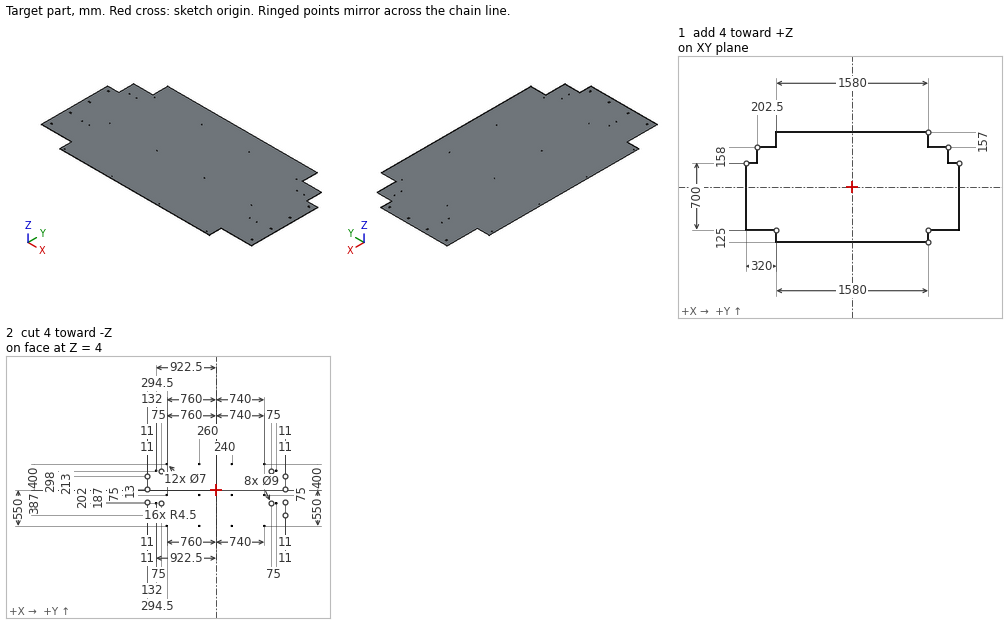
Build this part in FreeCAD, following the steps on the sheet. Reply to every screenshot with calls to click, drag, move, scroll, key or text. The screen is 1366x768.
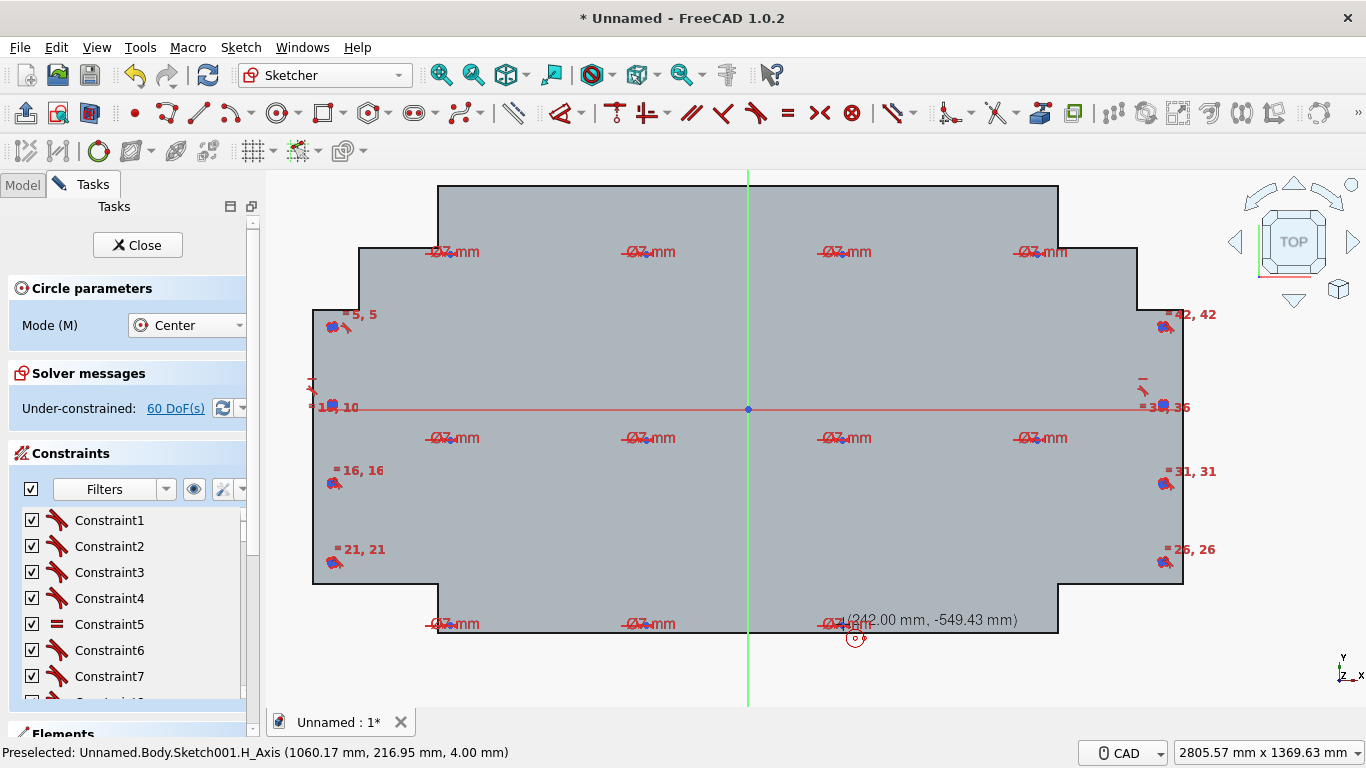
scroll(1038, 625, up, 15)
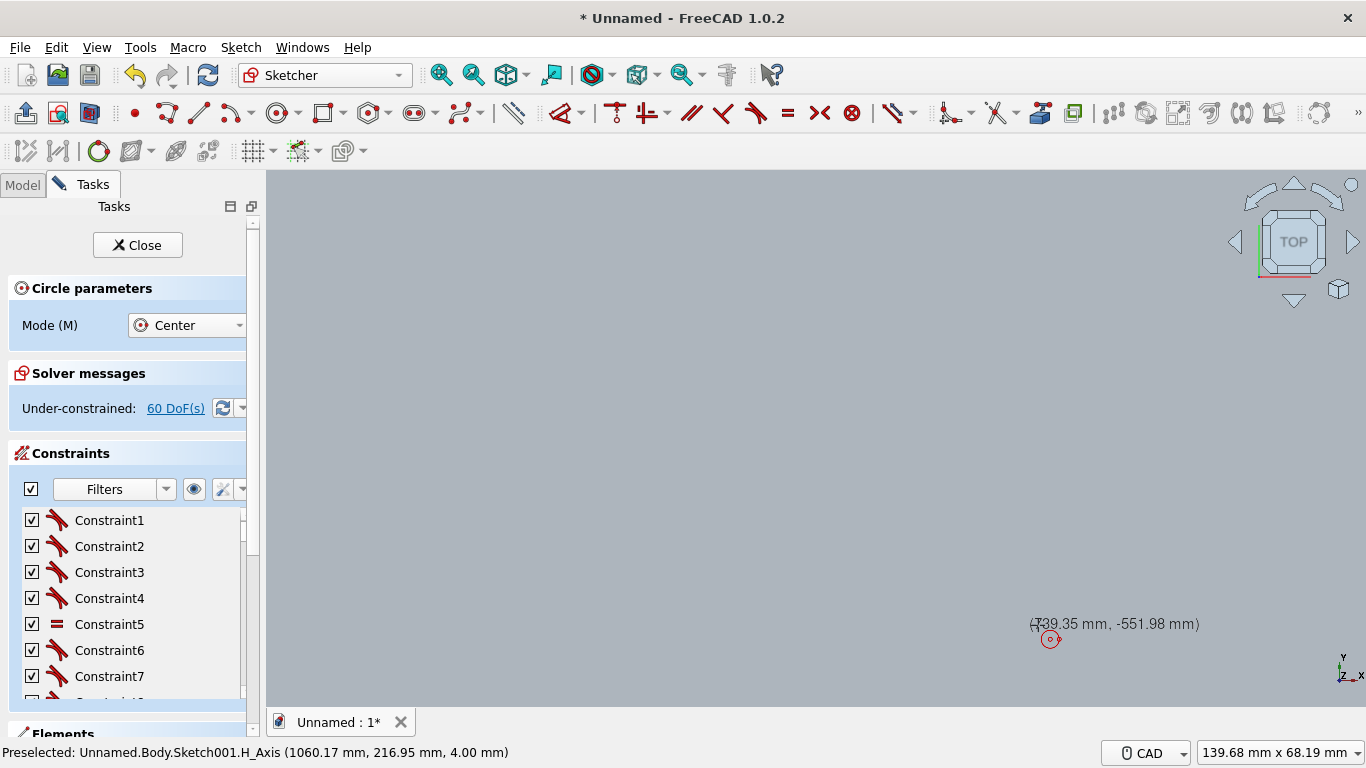
scroll(1038, 625, down, 15)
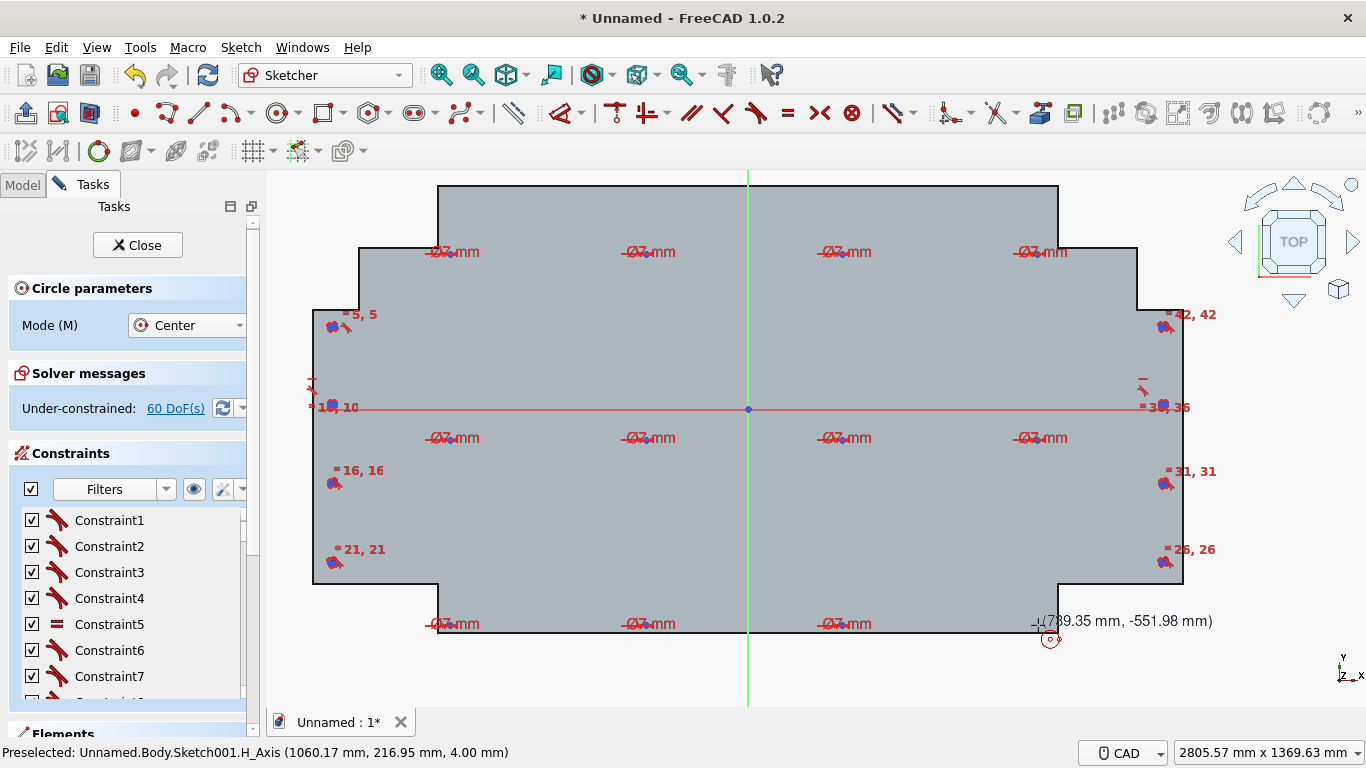
click(1038, 625)
move(1039, 624)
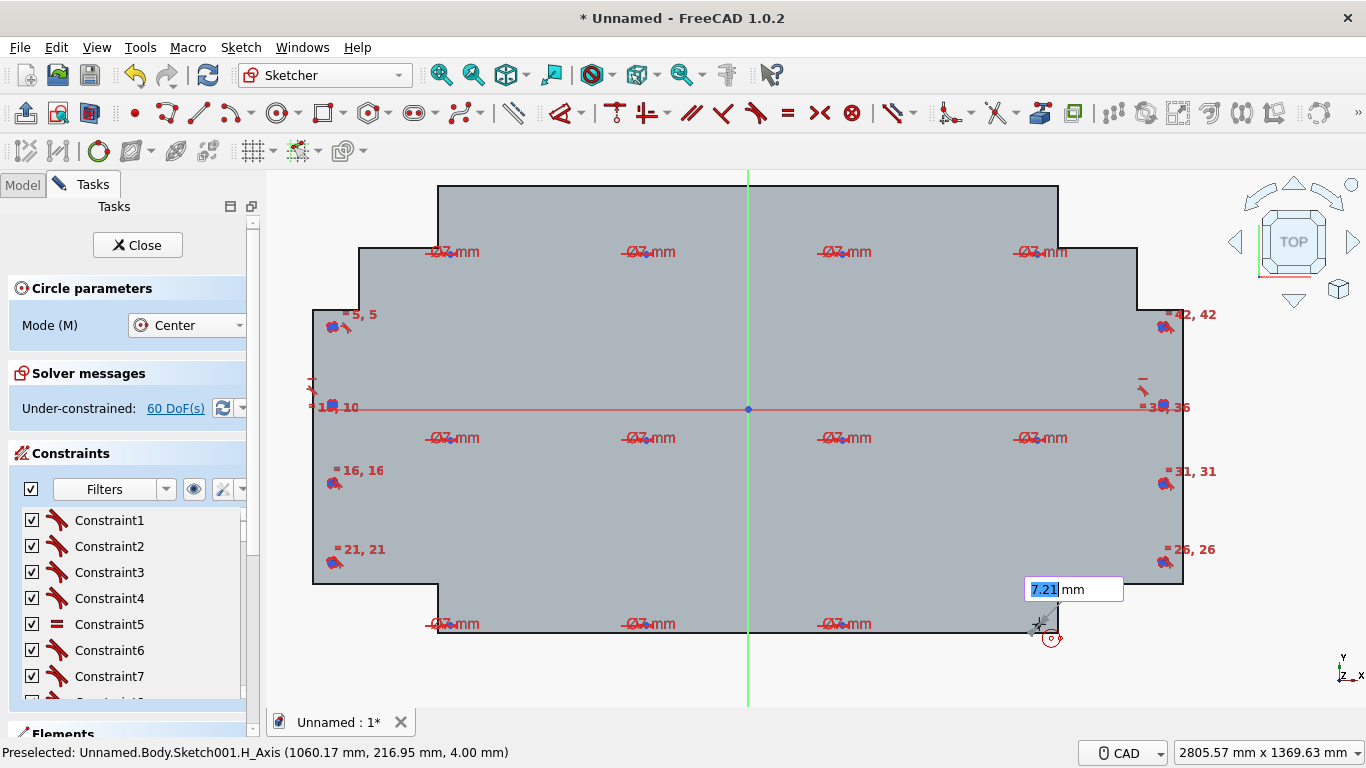
text(7)
key(Return)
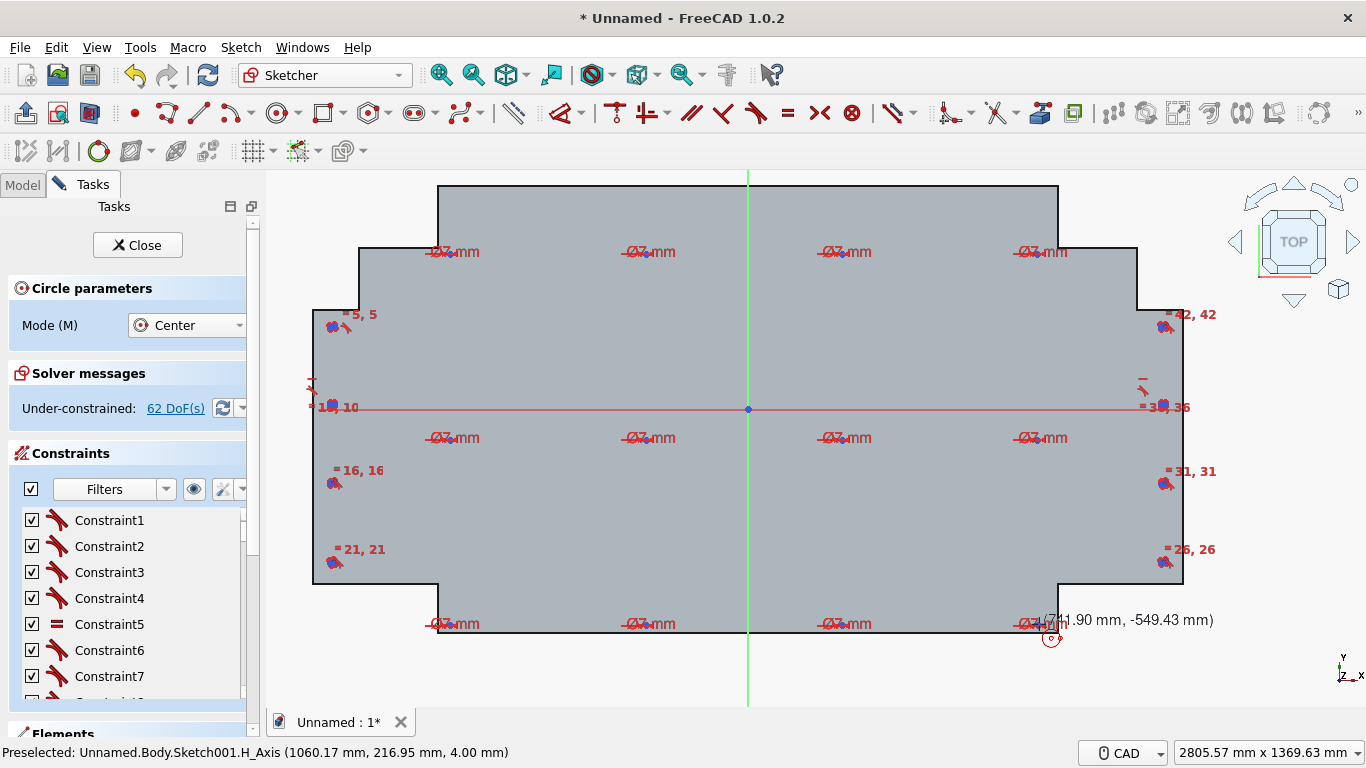
scroll(386, 293, up, 13)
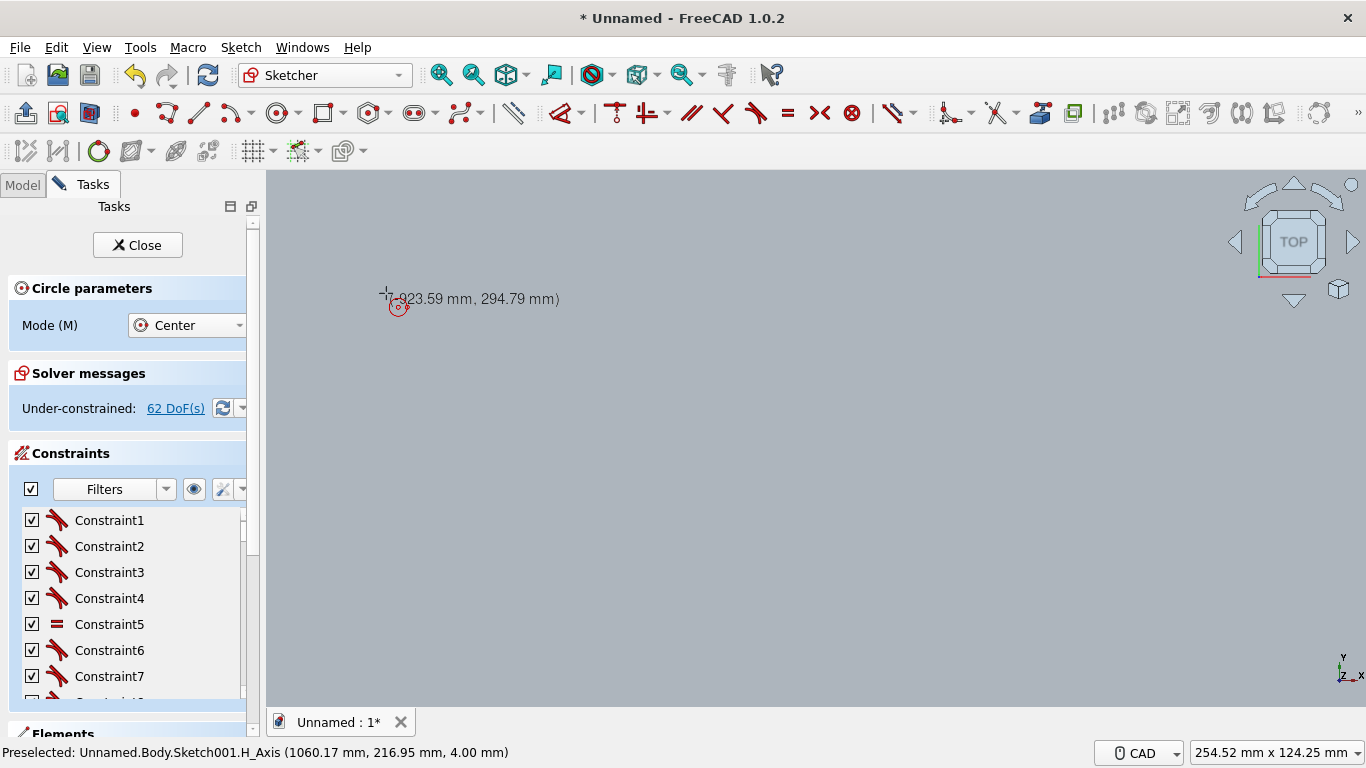
scroll(455, 321, down, 14)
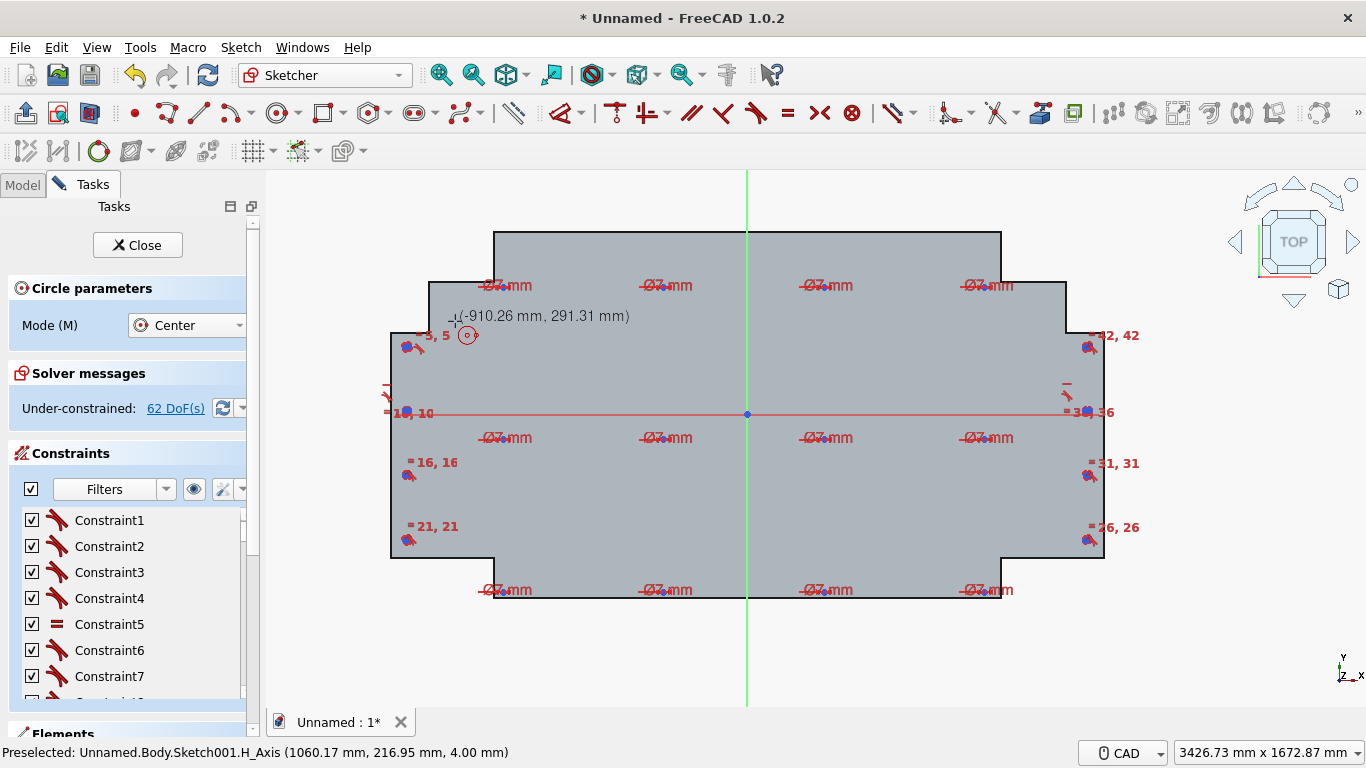
click(451, 319)
move(452, 318)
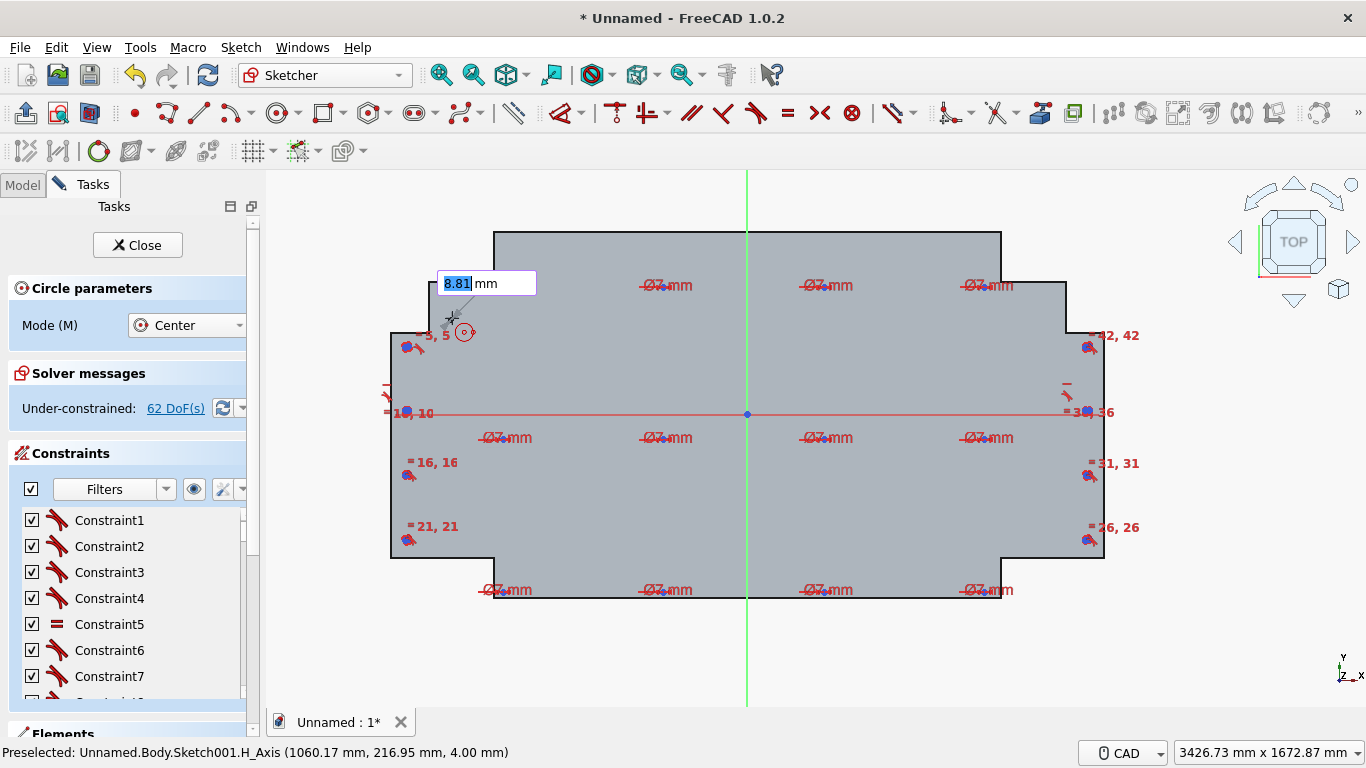
text(9)
key(Return)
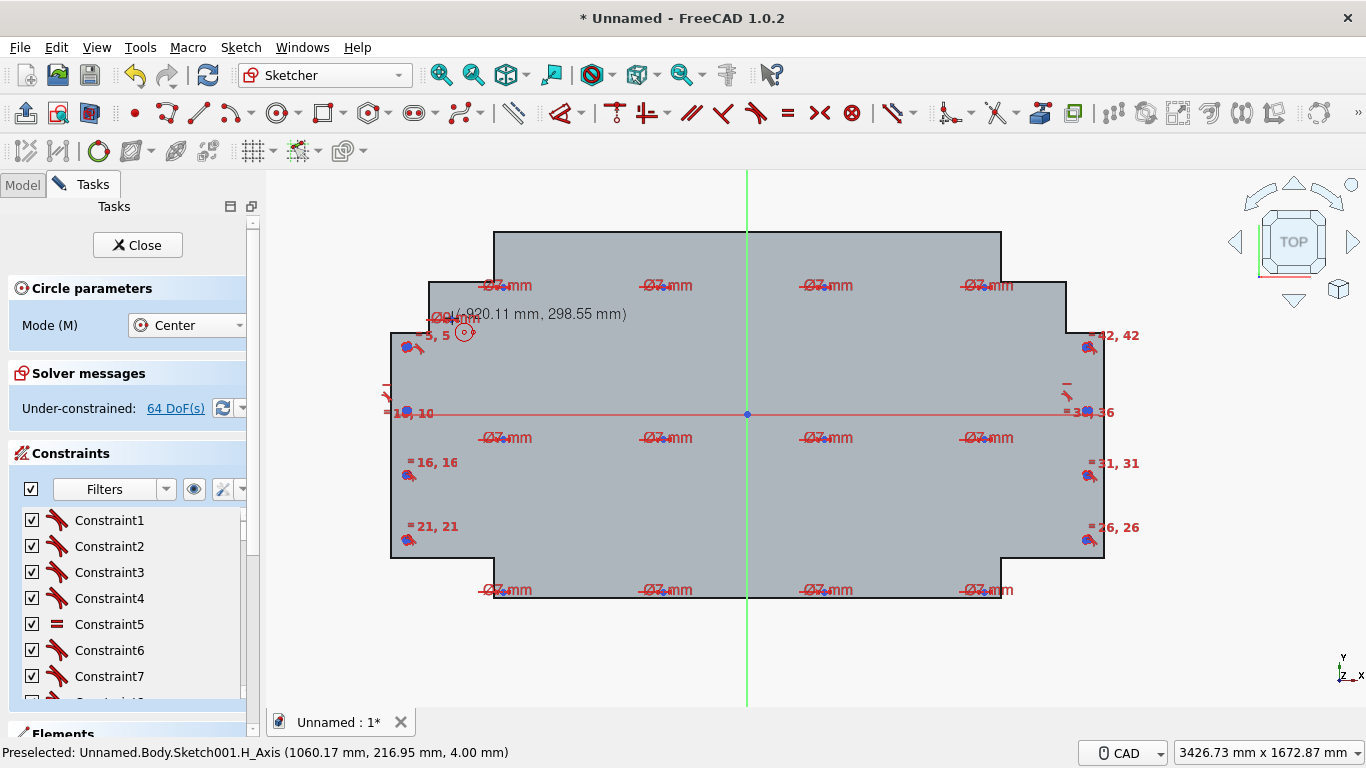
scroll(475, 319, up, 14)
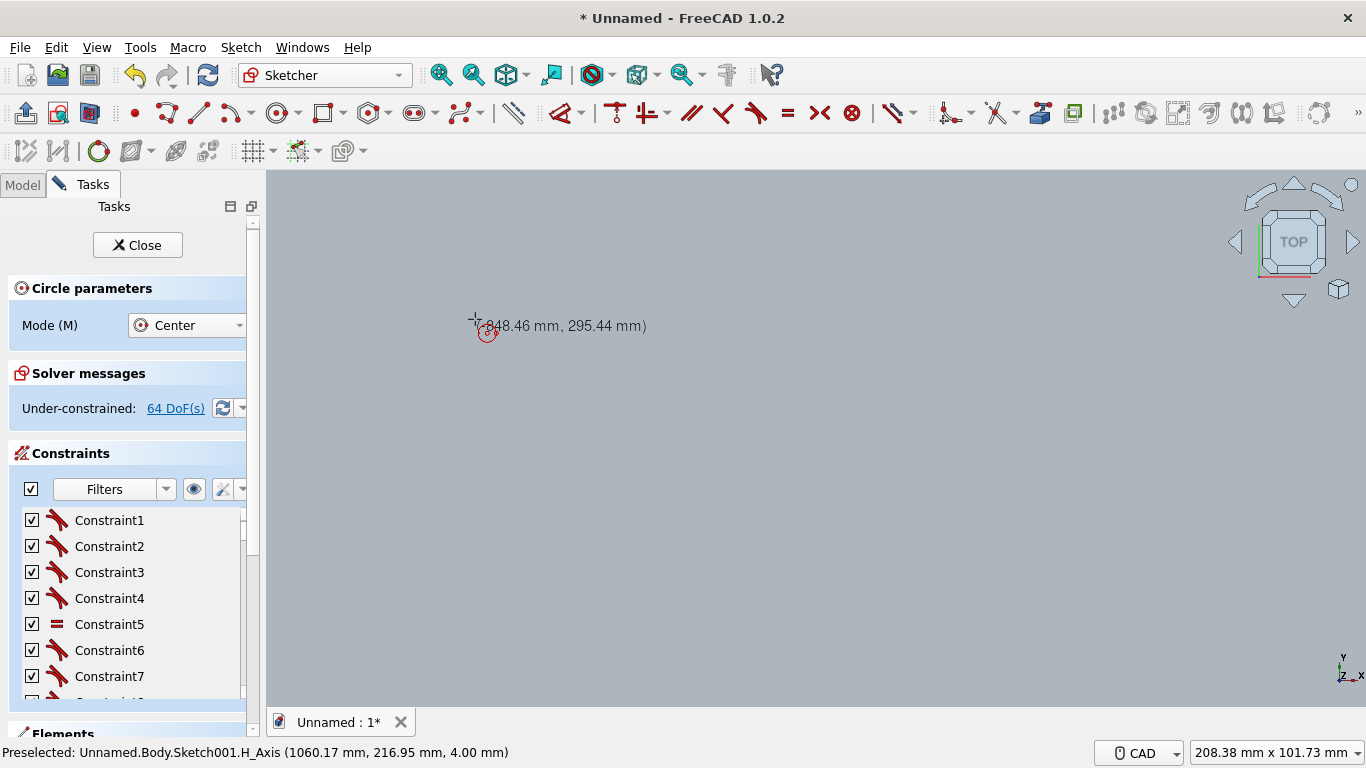
scroll(475, 319, down, 14)